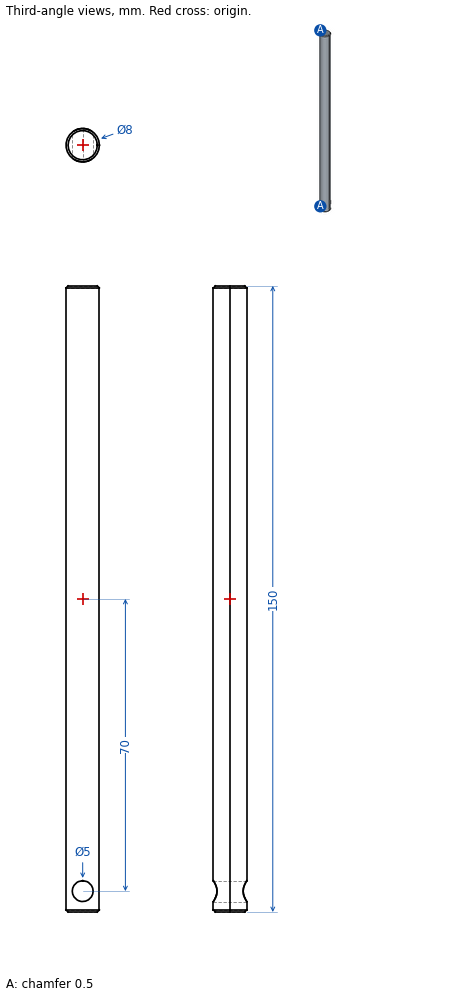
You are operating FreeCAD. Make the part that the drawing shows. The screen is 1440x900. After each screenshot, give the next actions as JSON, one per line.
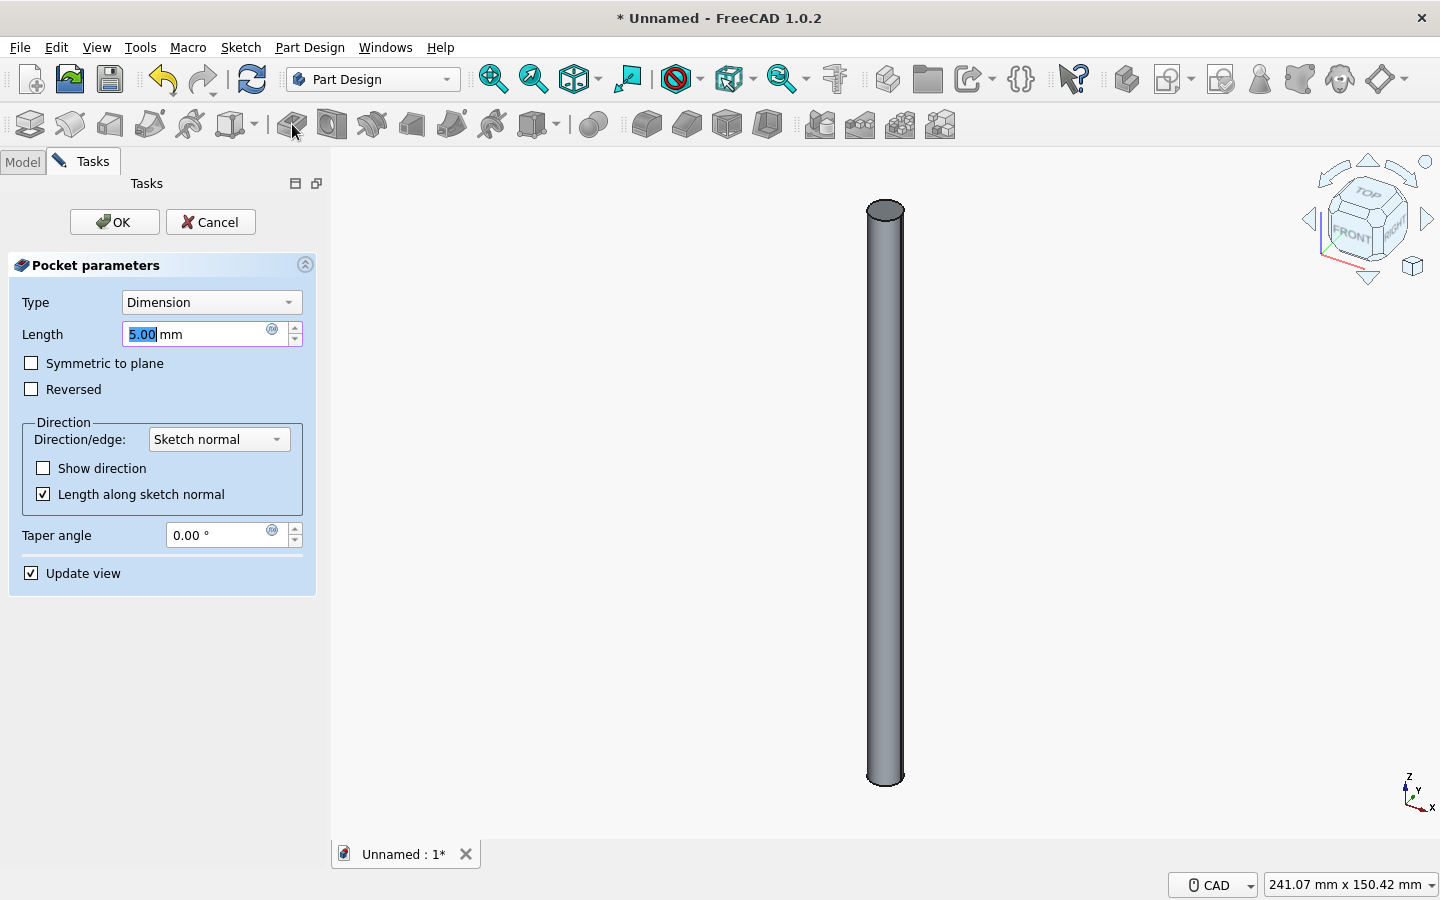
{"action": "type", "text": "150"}
{"action": "key", "text": "Tab"}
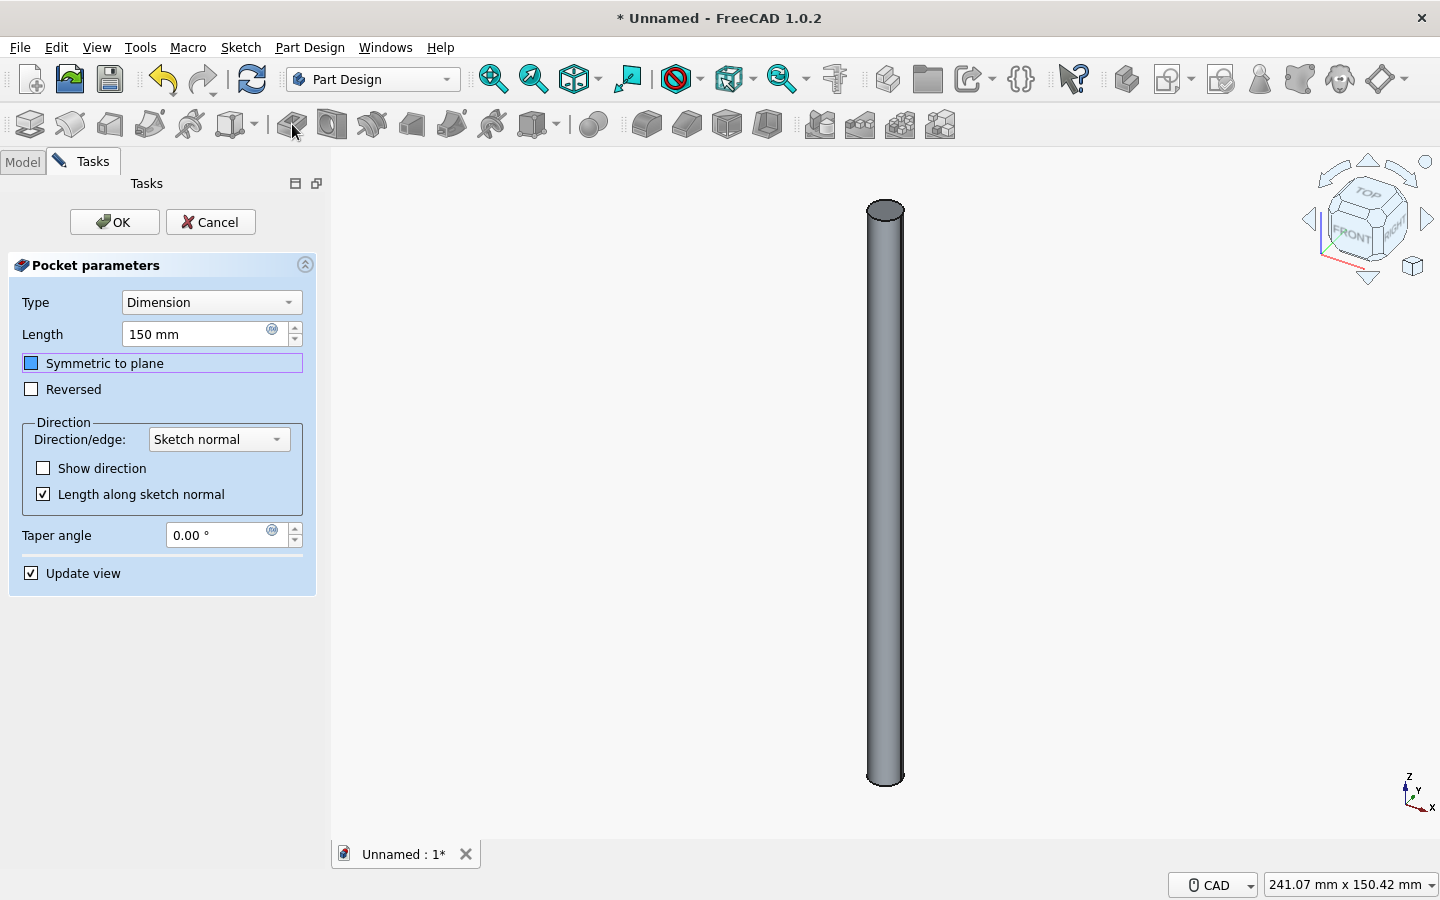
{"action": "left_click", "coordinate": [30, 363]}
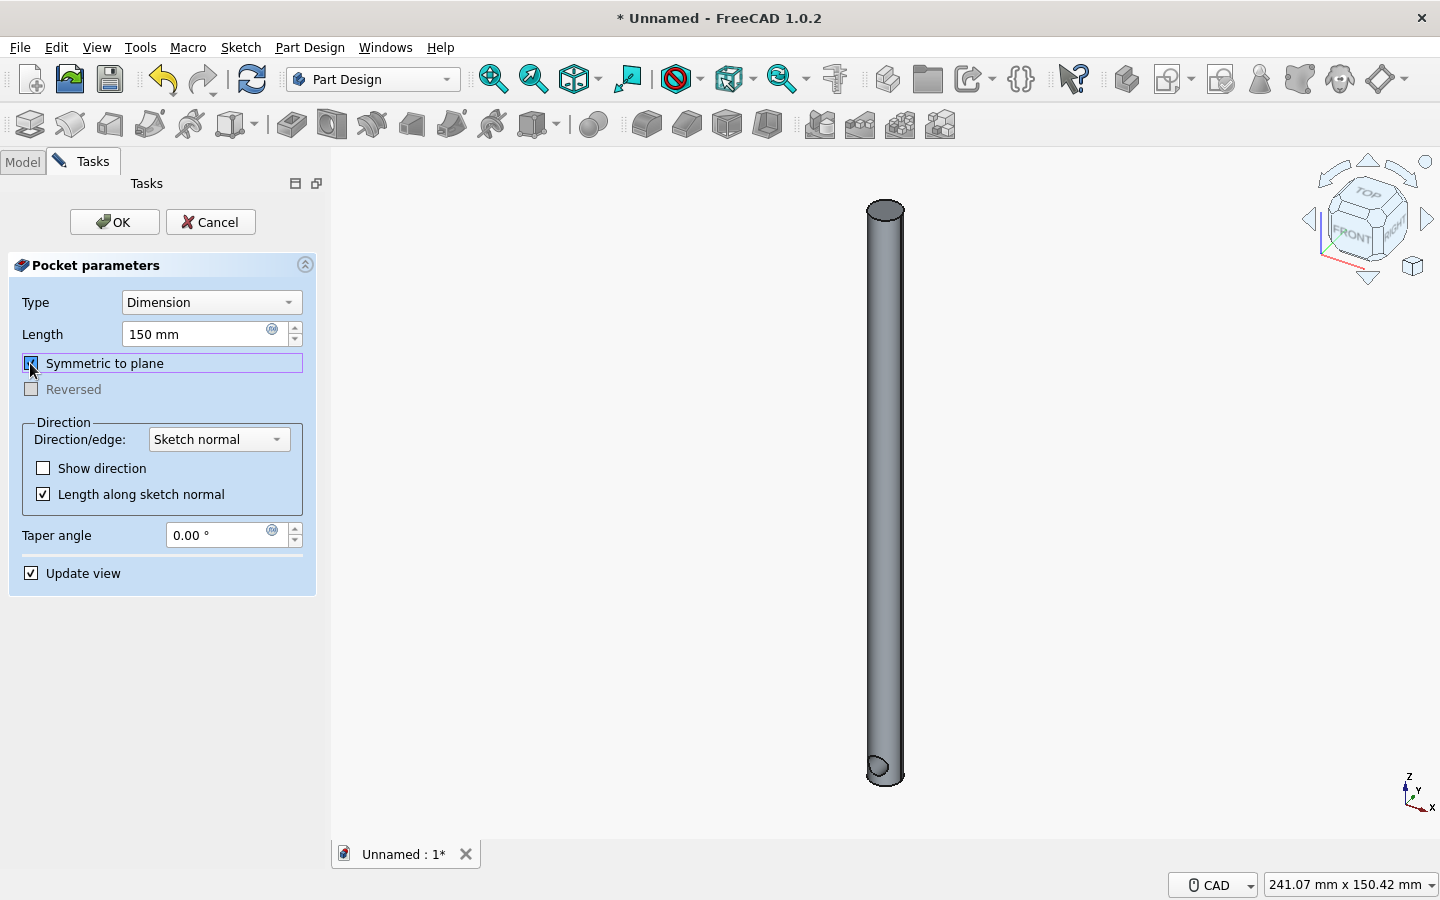
{"action": "left_click", "coordinate": [115, 222]}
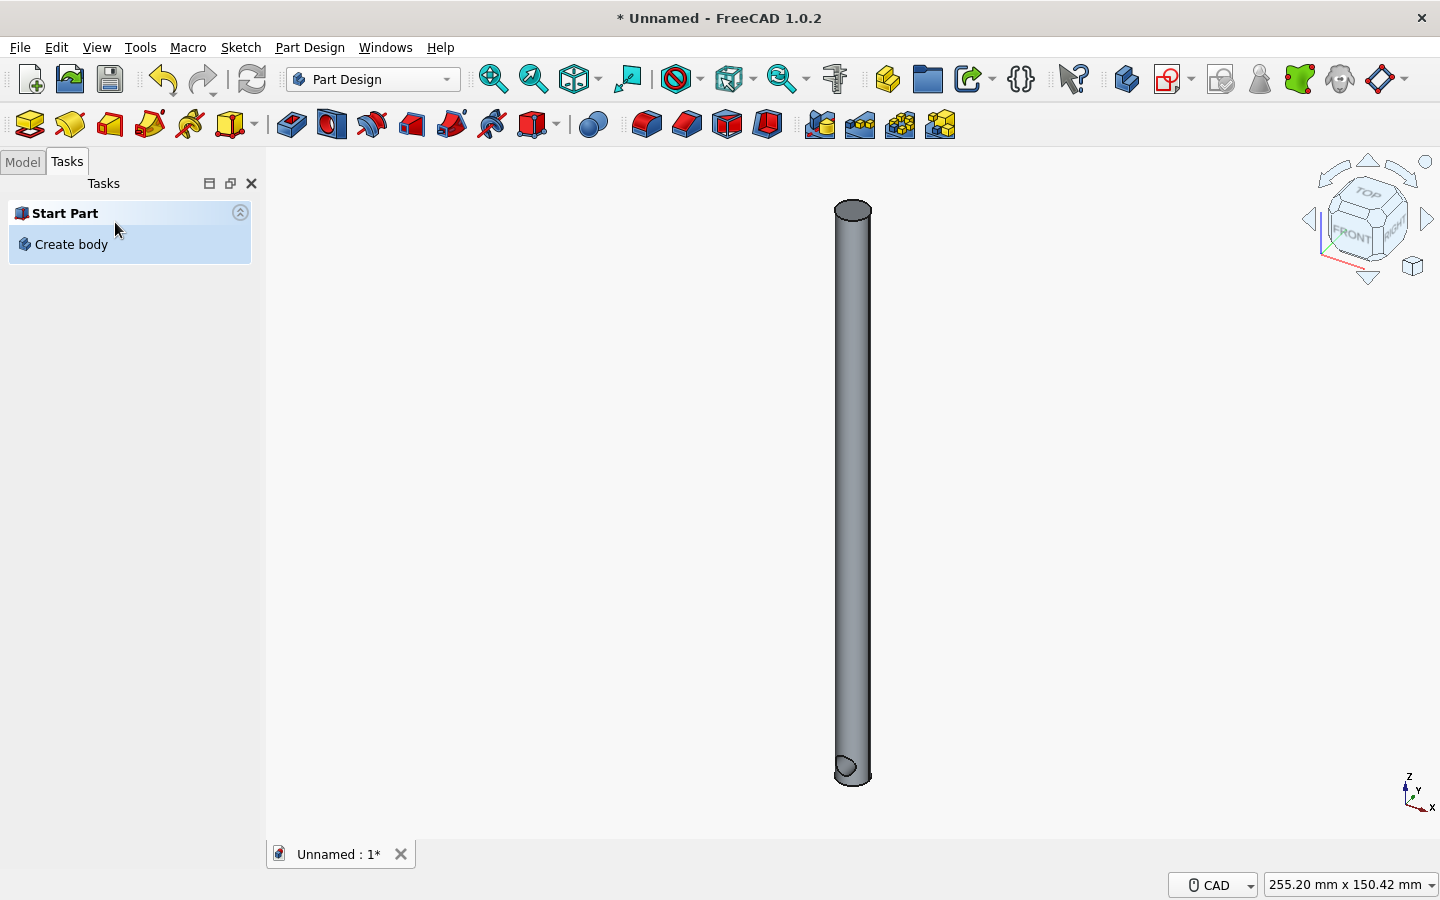
{"action": "left_click", "coordinate": [839, 782]}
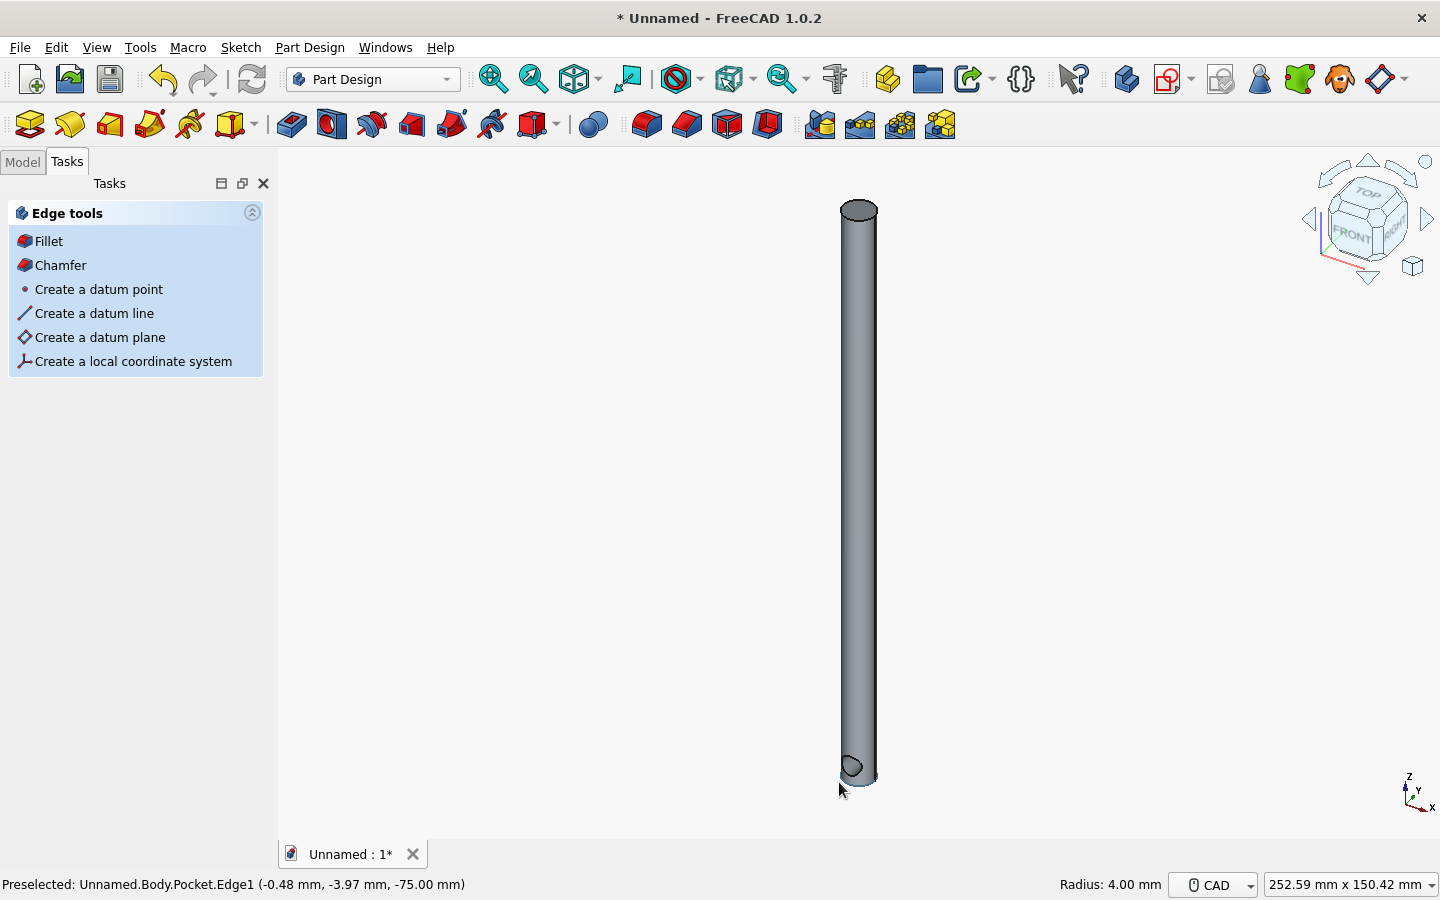
{"action": "left_click", "coordinate": [843, 204], "text": "ctrl"}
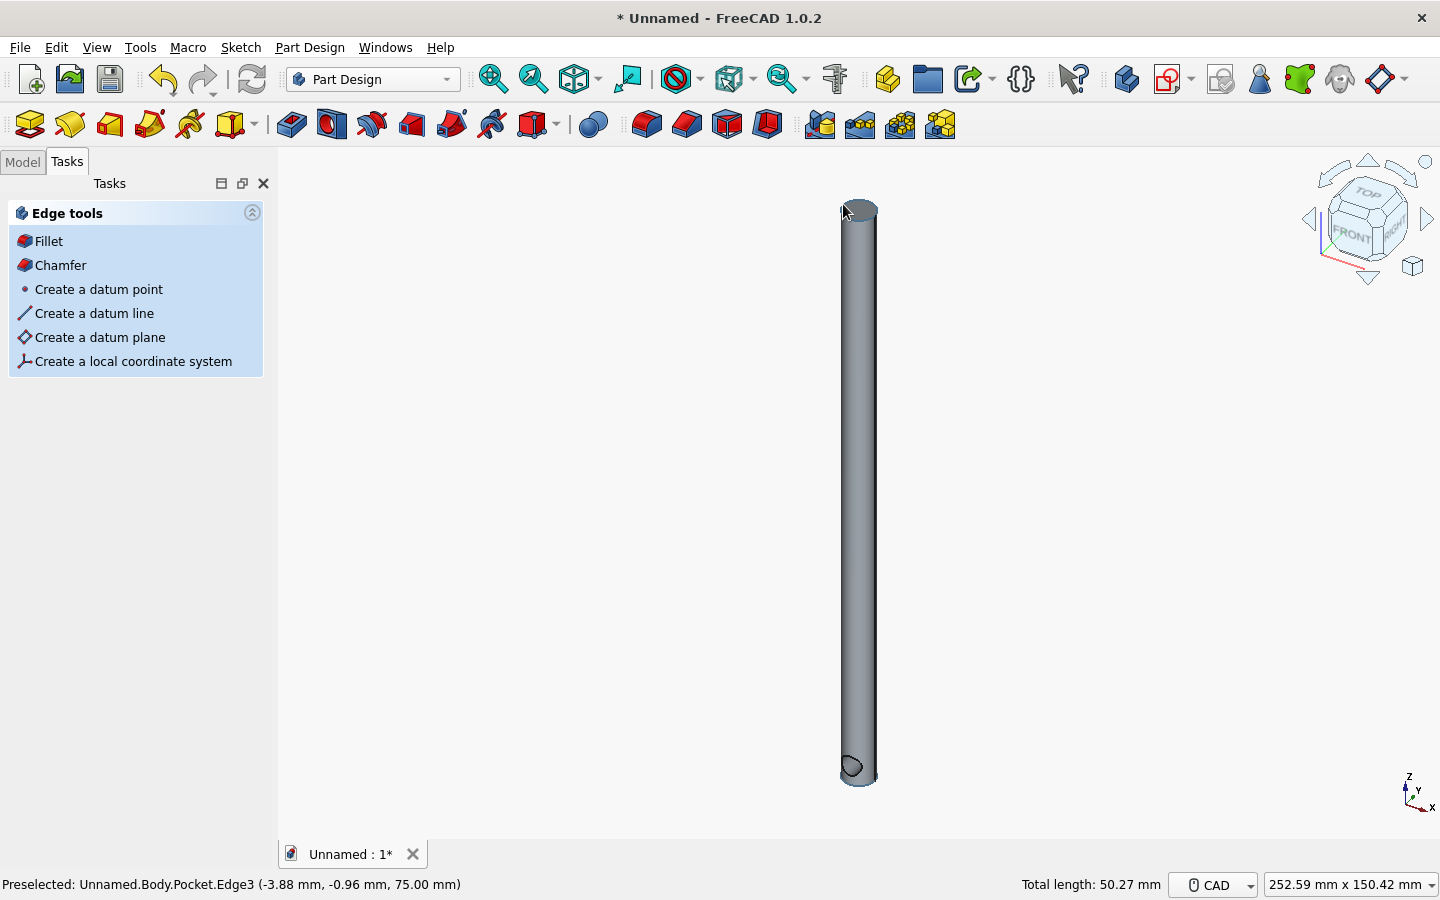
{"action": "left_click", "coordinate": [688, 124]}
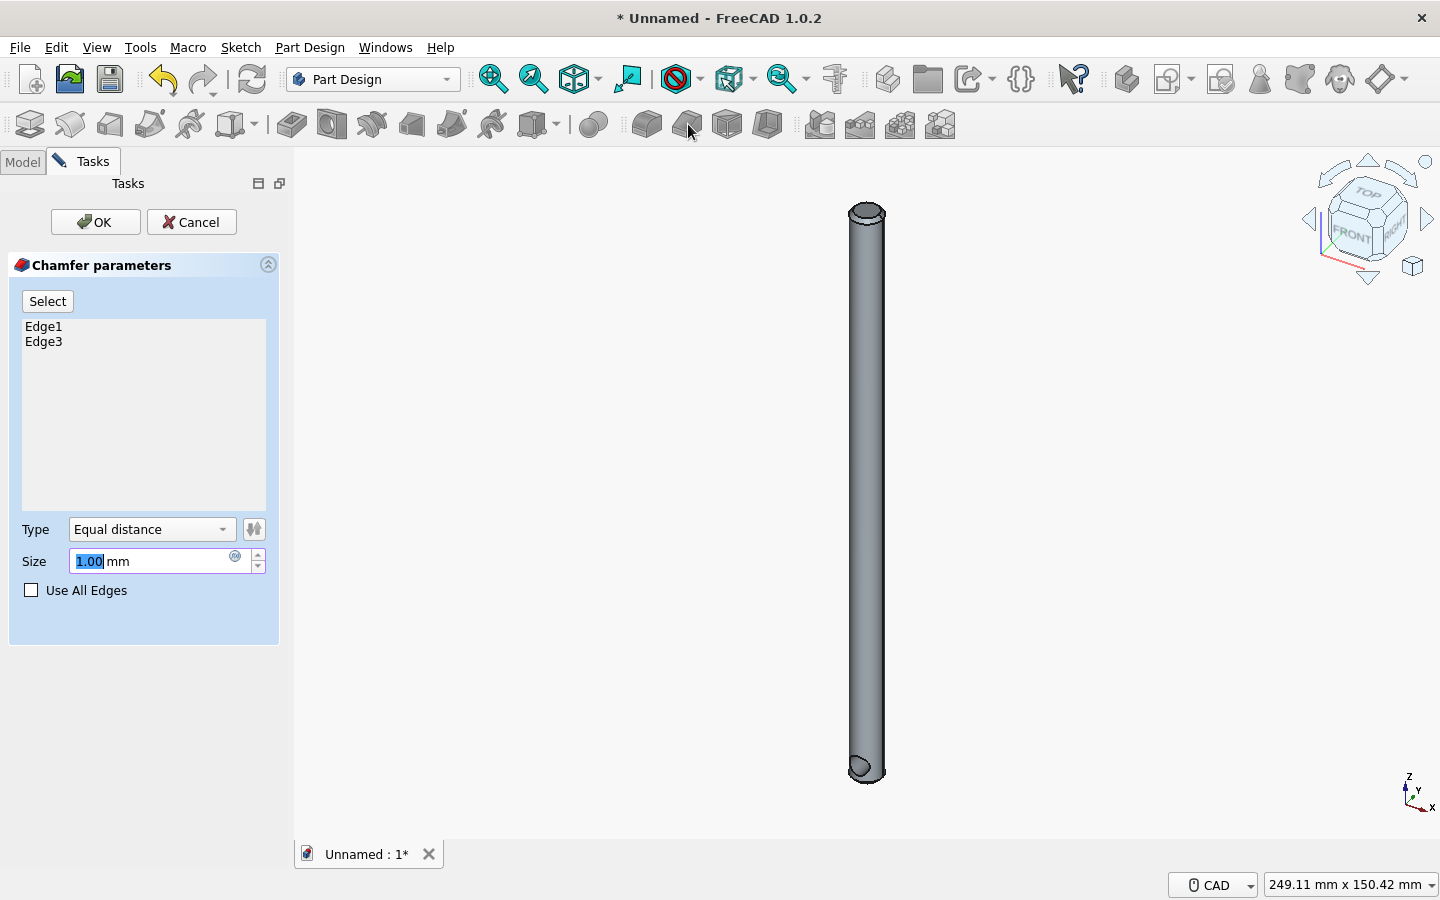
{"action": "type", "text": "0.5"}
{"action": "key", "text": "Tab"}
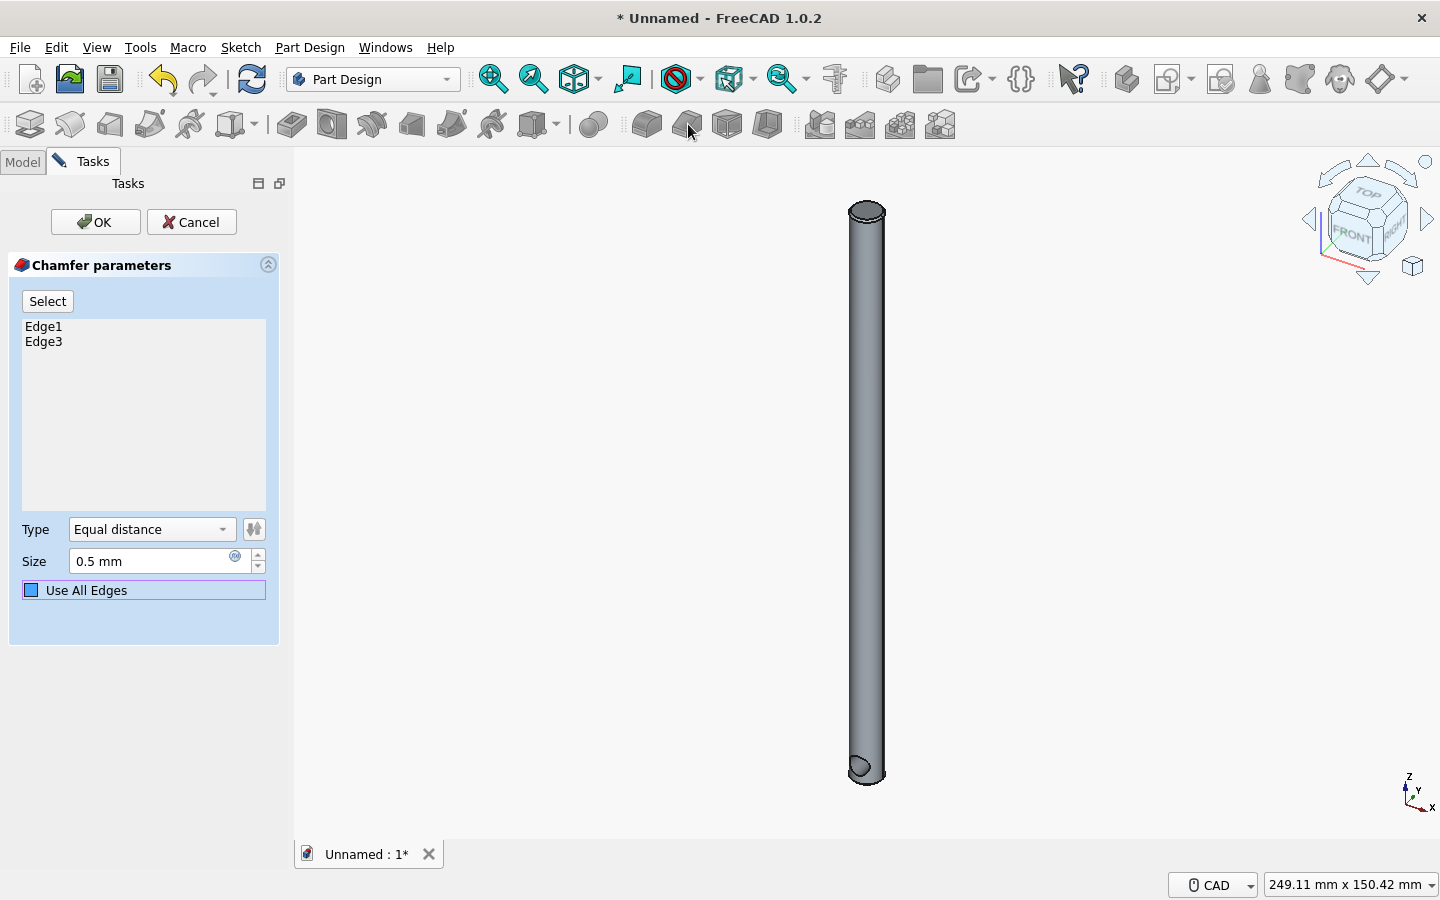
{"action": "left_click", "coordinate": [96, 222]}